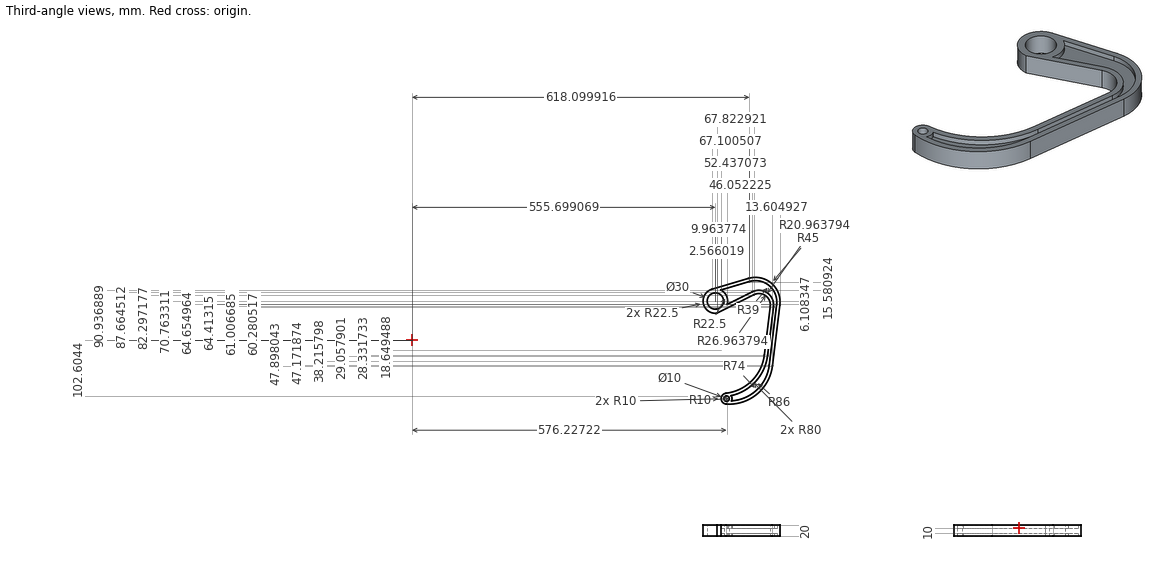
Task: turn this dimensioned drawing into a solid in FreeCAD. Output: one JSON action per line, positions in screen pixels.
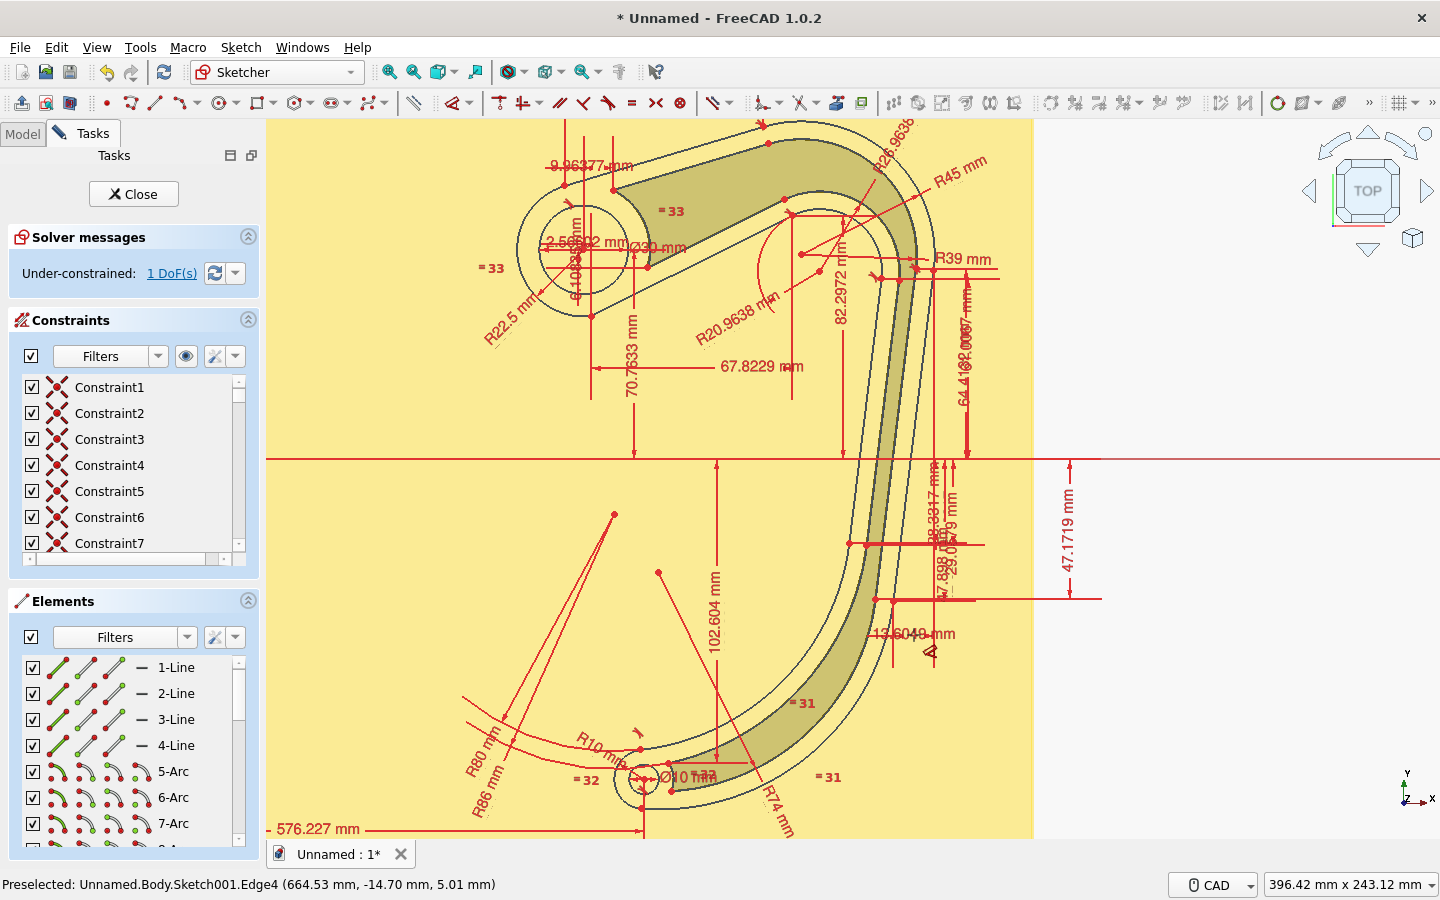
{"action": "left_click", "coordinate": [584, 250]}
{"action": "left_click", "coordinate": [439, 216]}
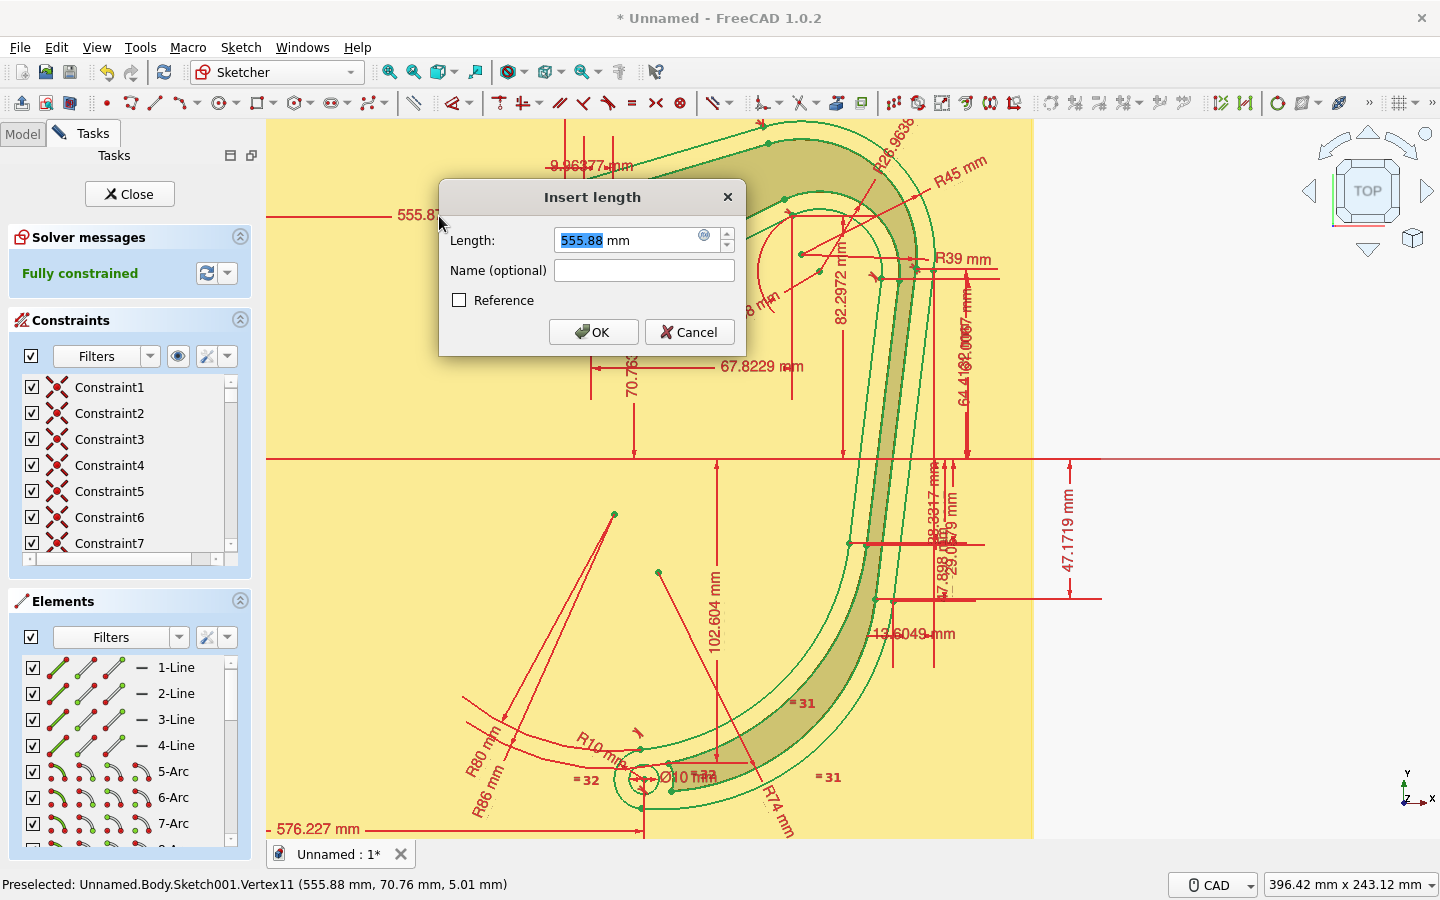
{"action": "type", "text": "555.699069"}
{"action": "key", "text": "Return"}
{"action": "key", "text": "Escape"}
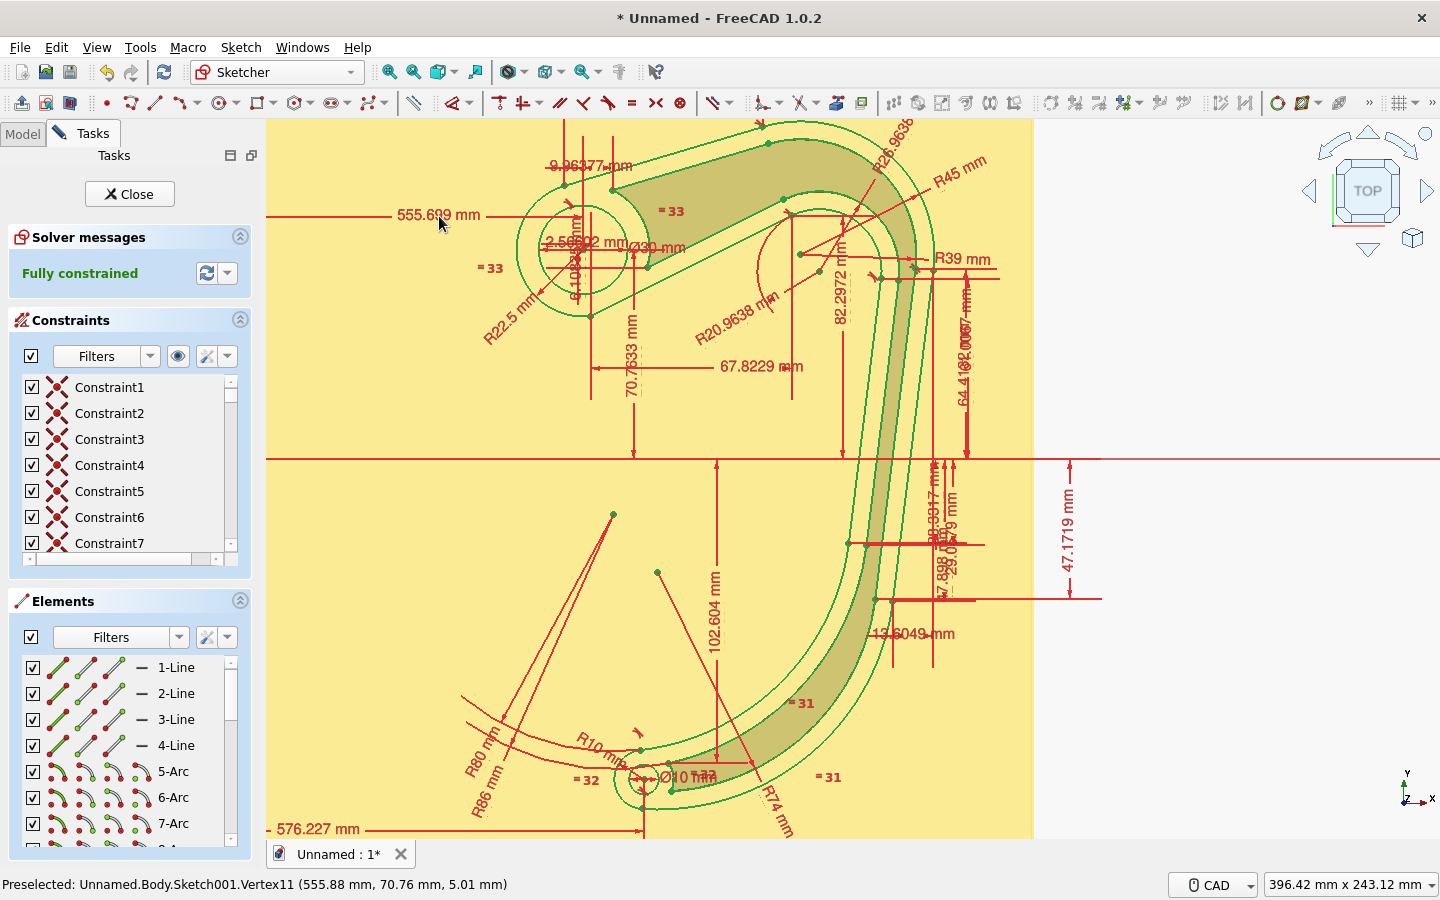
{"action": "left_click", "coordinate": [130, 194]}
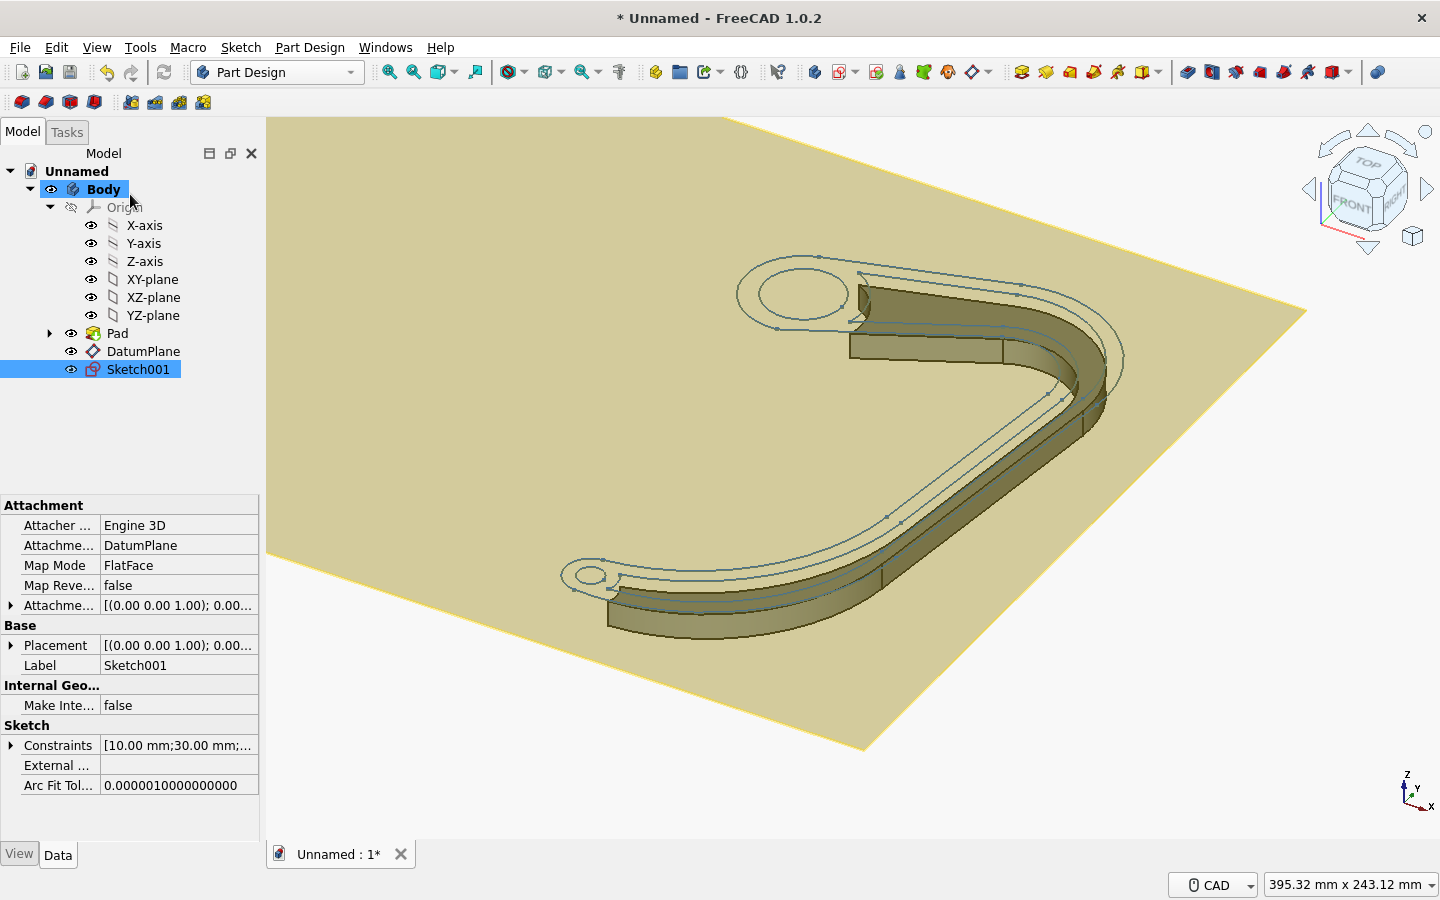
{"action": "left_click", "coordinate": [1022, 72]}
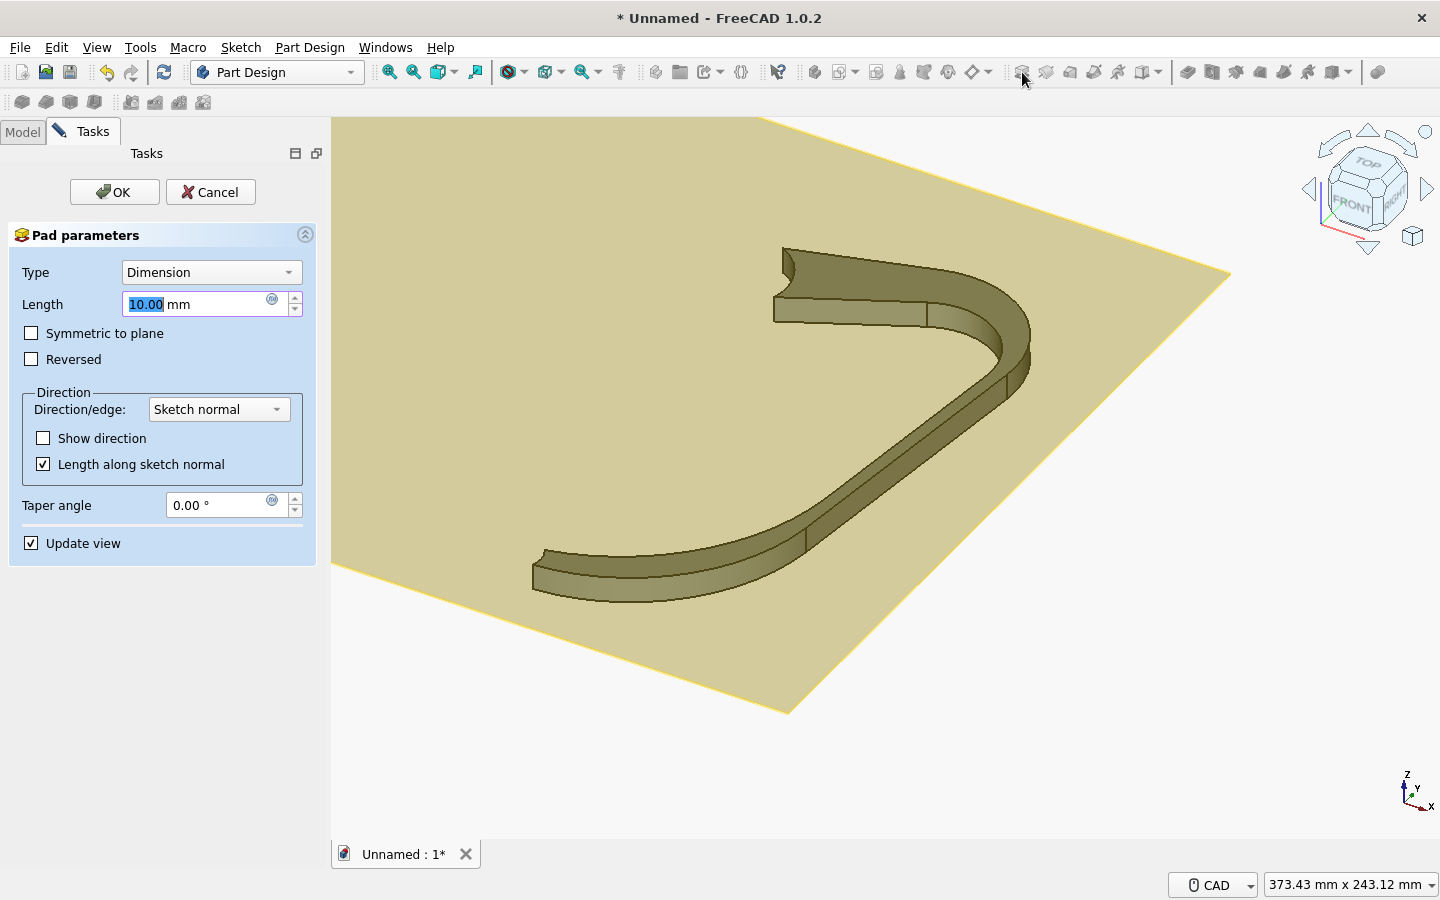
{"action": "type", "text": "20"}
{"action": "key", "text": "Tab"}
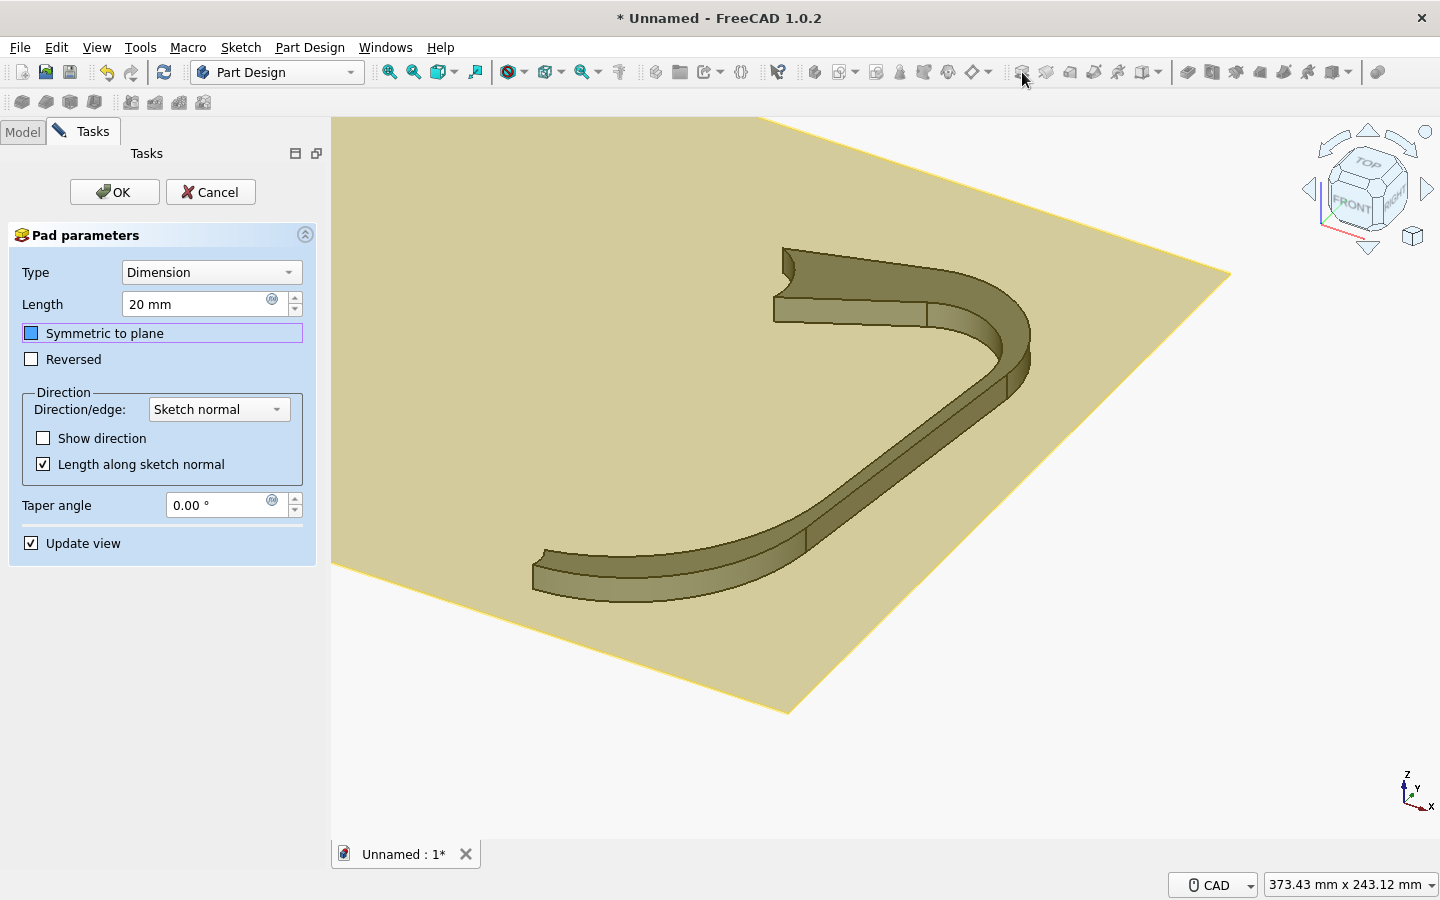
{"action": "left_click", "coordinate": [30, 359]}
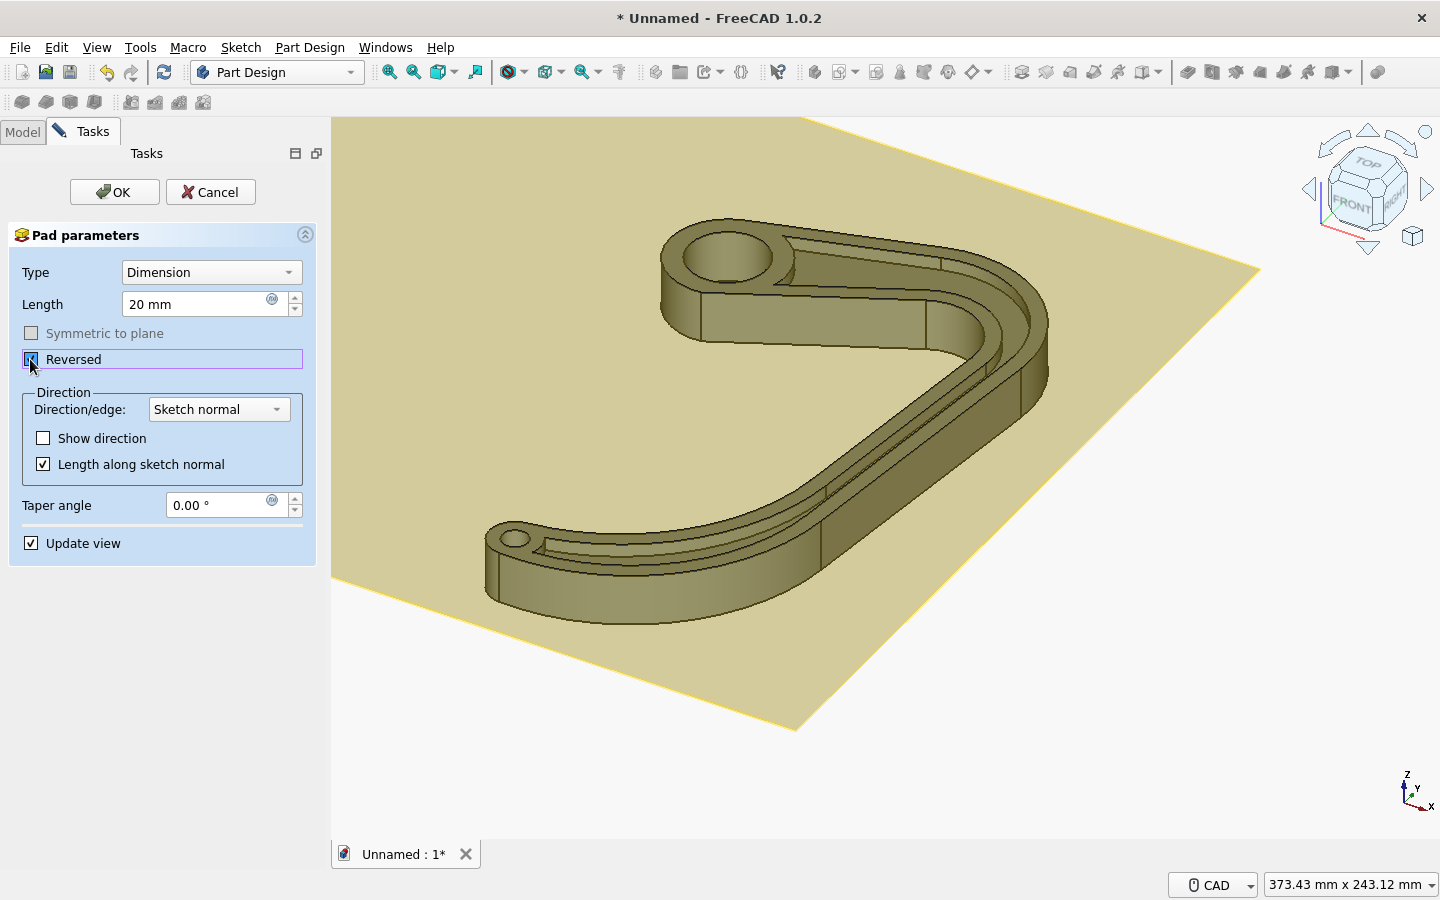
{"action": "left_click", "coordinate": [115, 192]}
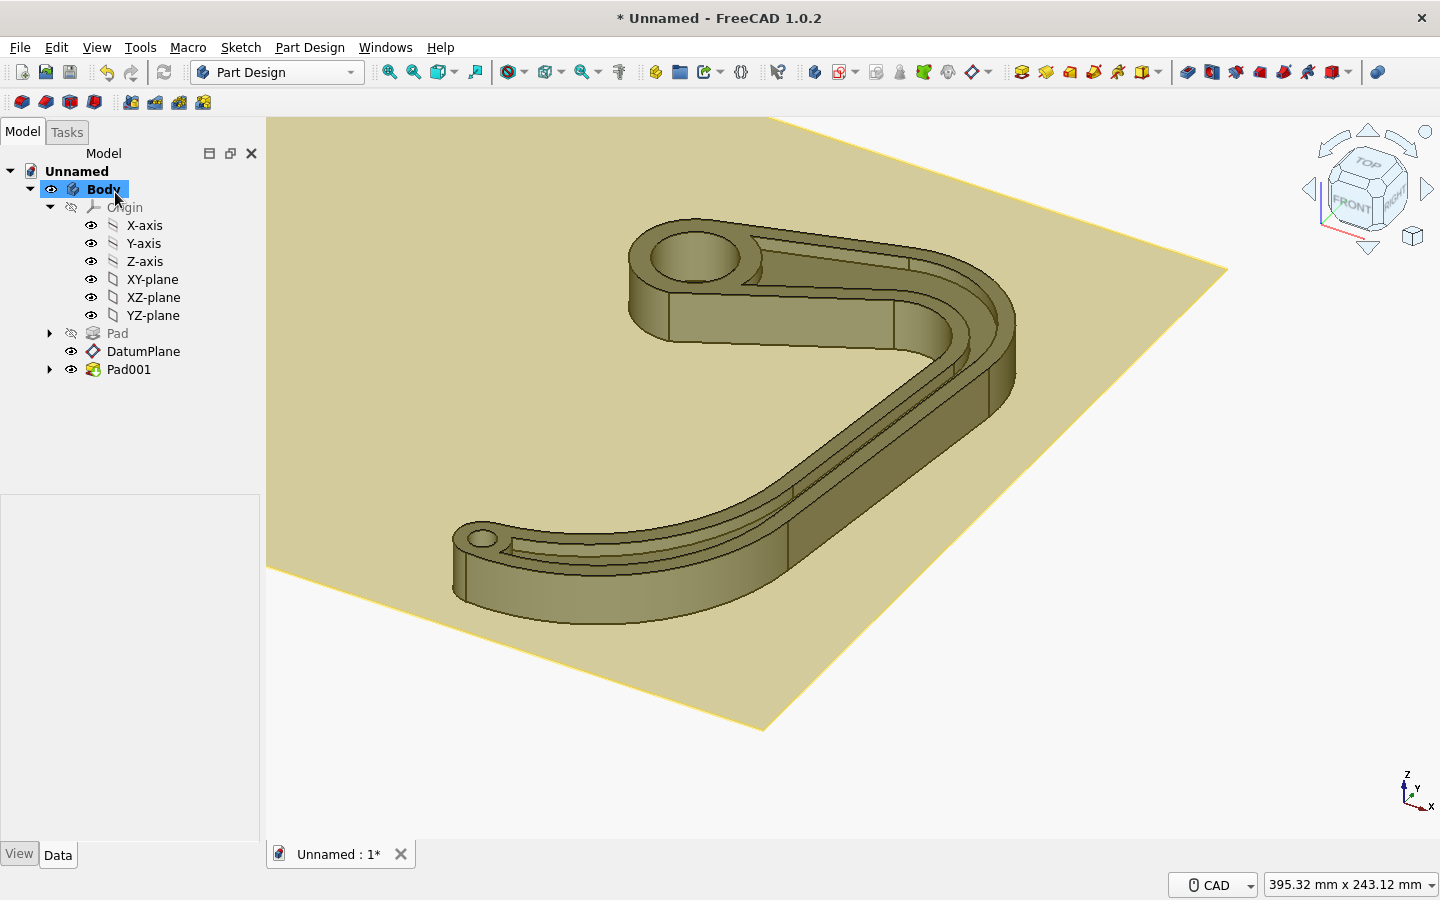
{"action": "left_click", "coordinate": [116, 351]}
{"action": "key", "text": "space"}